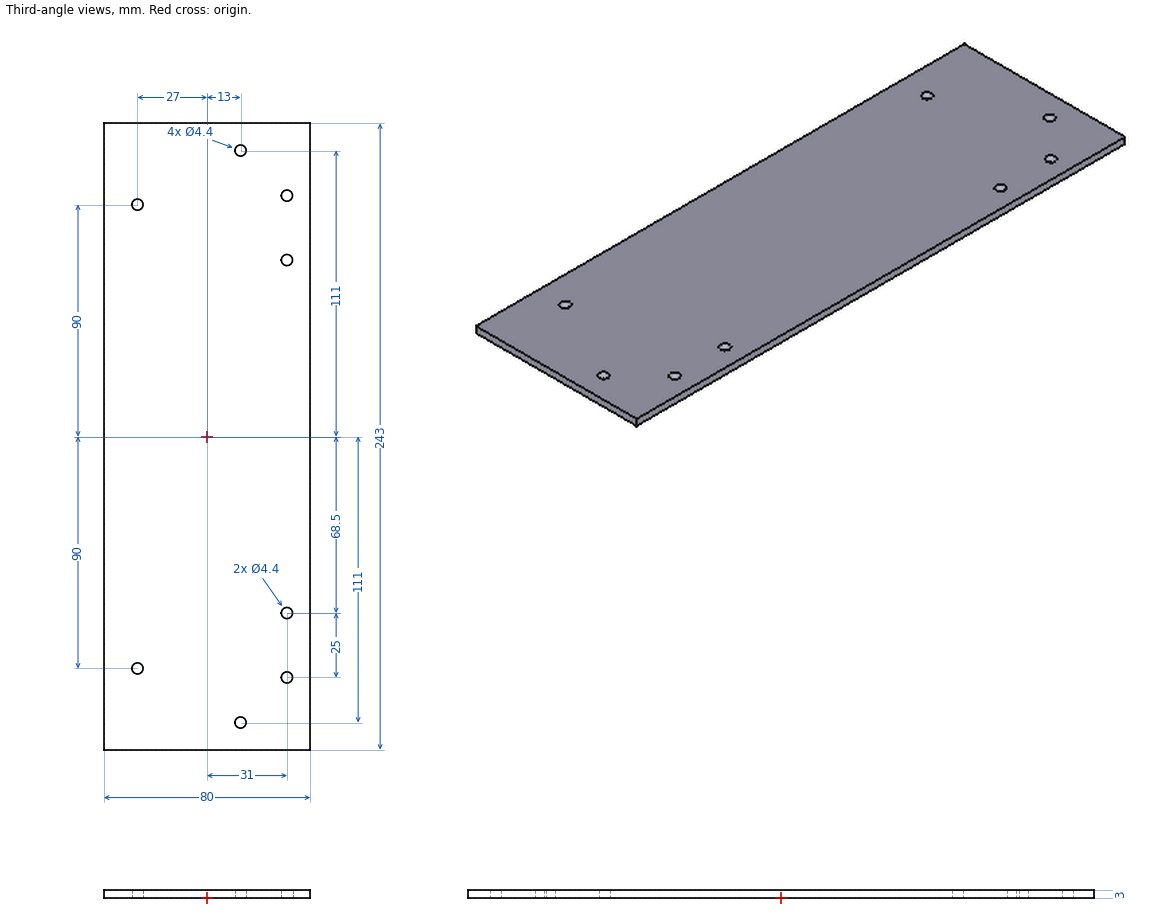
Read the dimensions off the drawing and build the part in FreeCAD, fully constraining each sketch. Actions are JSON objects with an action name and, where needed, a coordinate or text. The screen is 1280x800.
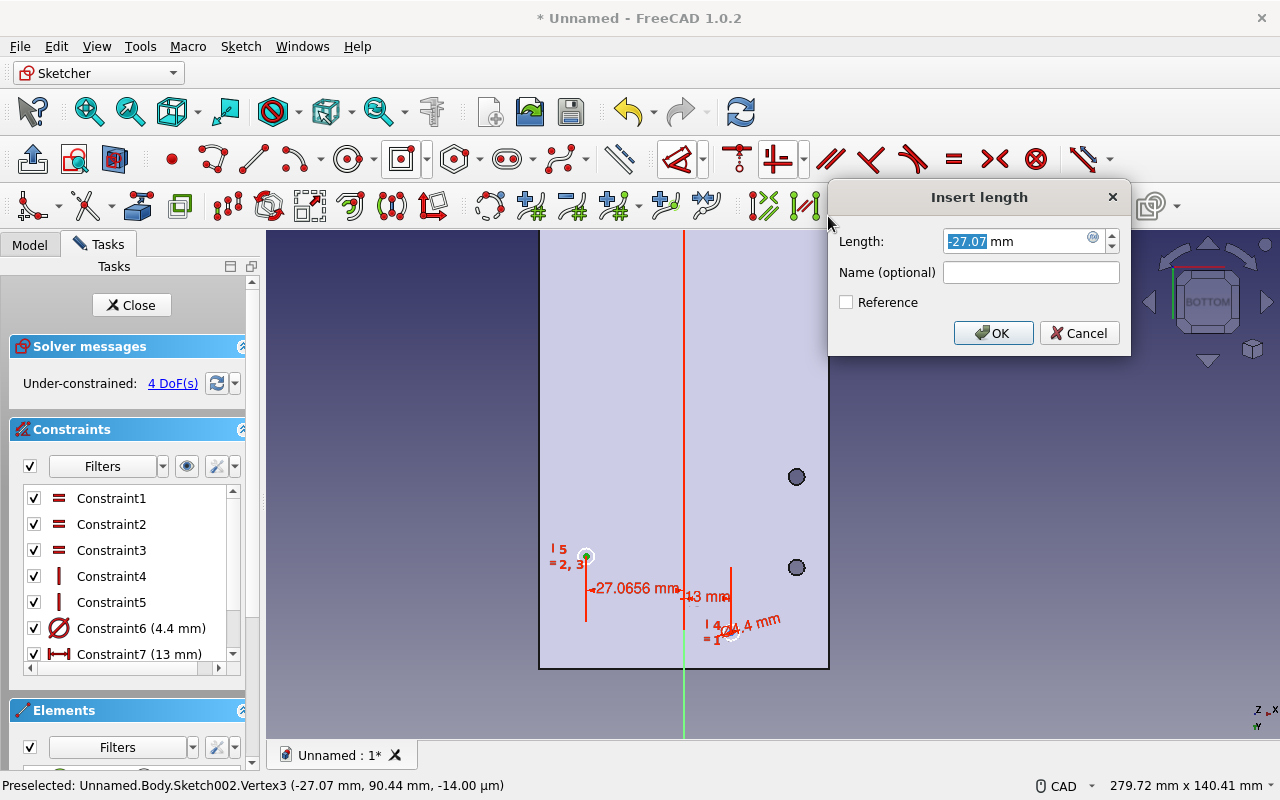
{"action": "type", "text": "-27"}
{"action": "key", "text": "Return"}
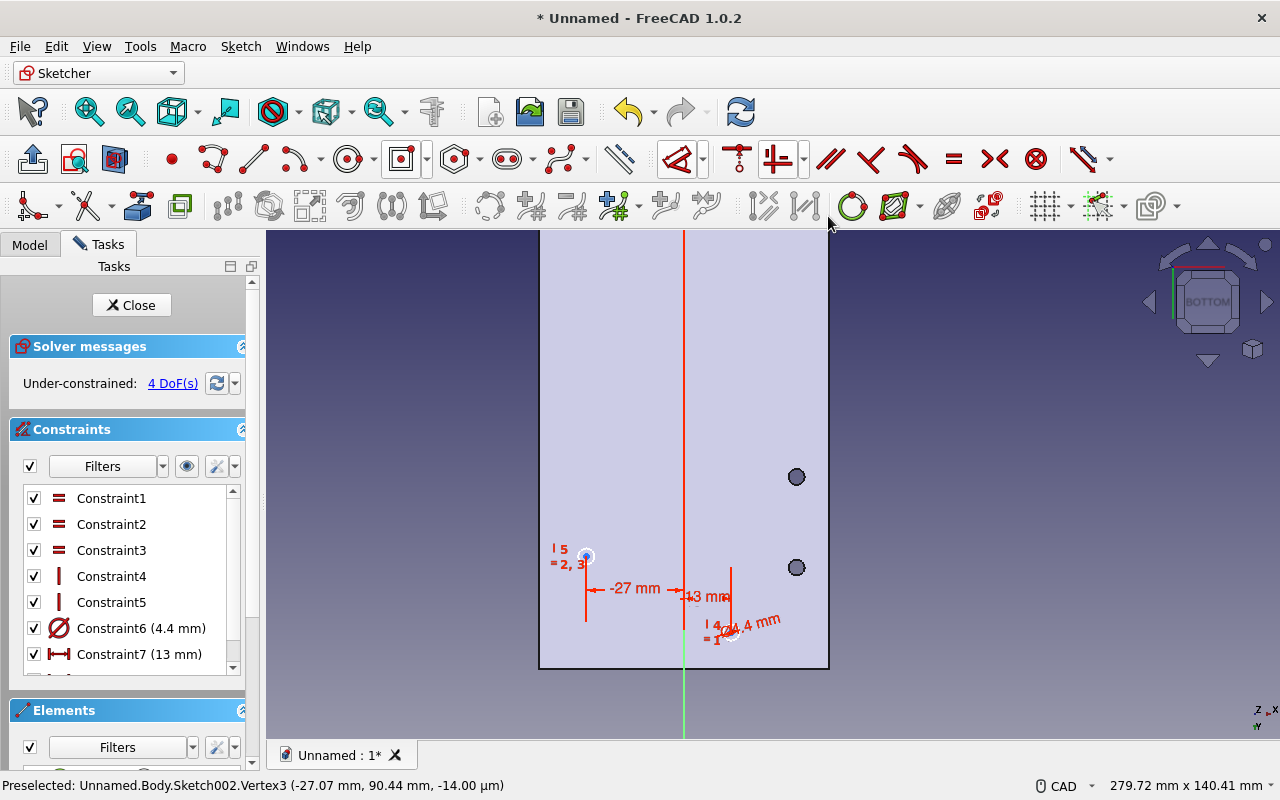
{"action": "left_click", "coordinate": [586, 556]}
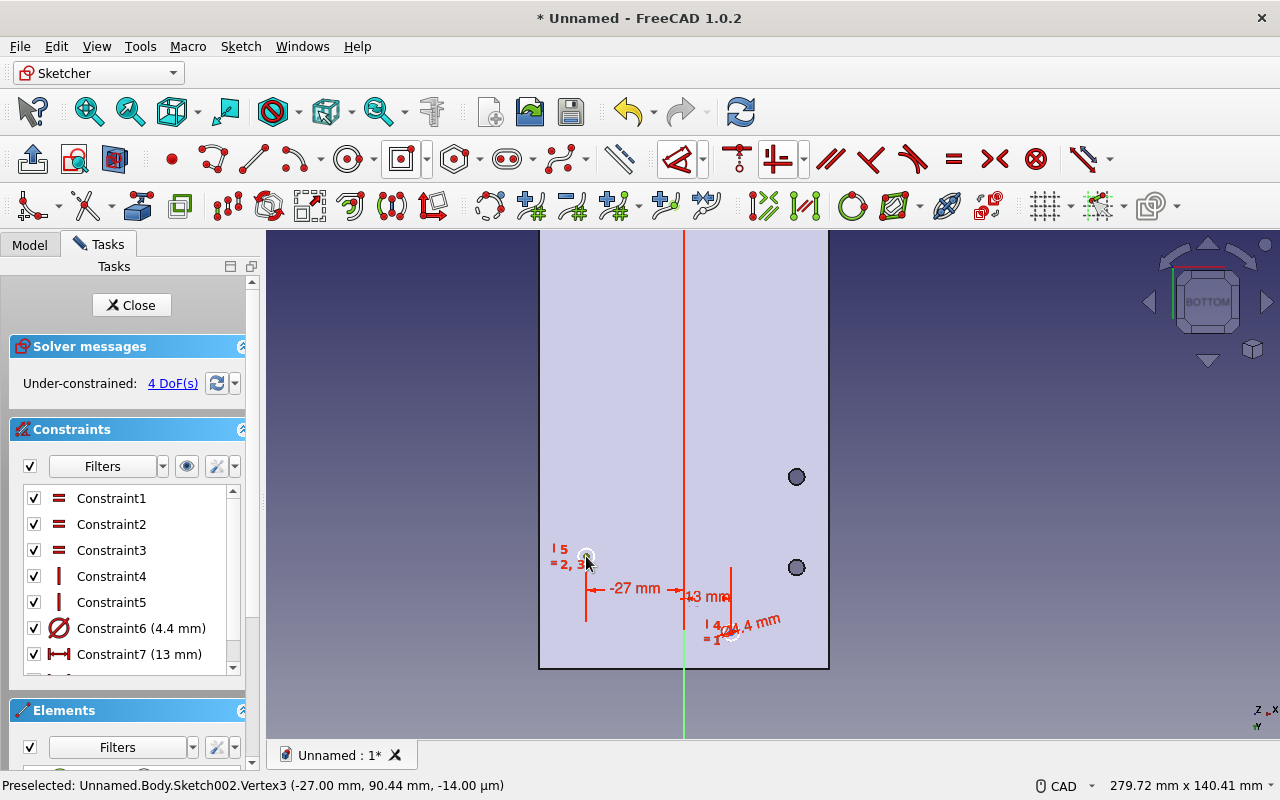
{"action": "key", "text": "i"}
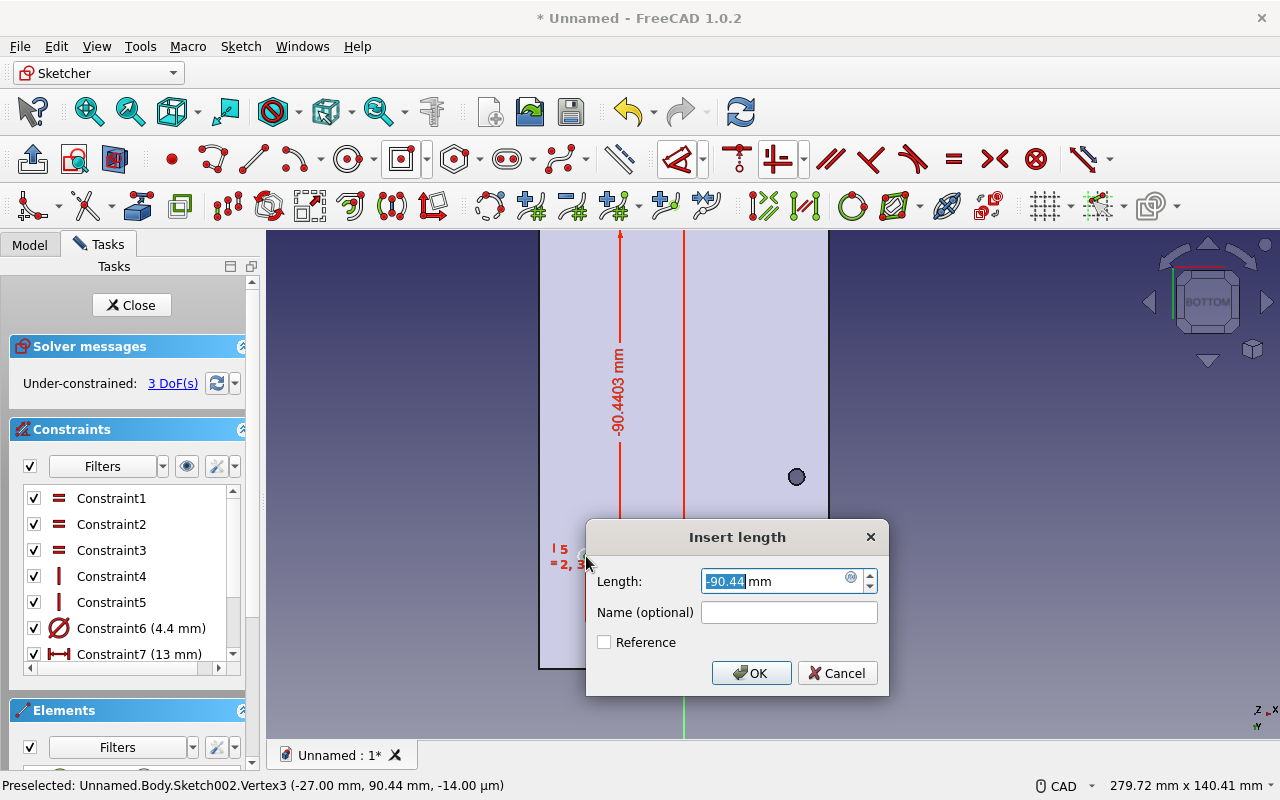
{"action": "type", "text": "-90"}
{"action": "key", "text": "Return"}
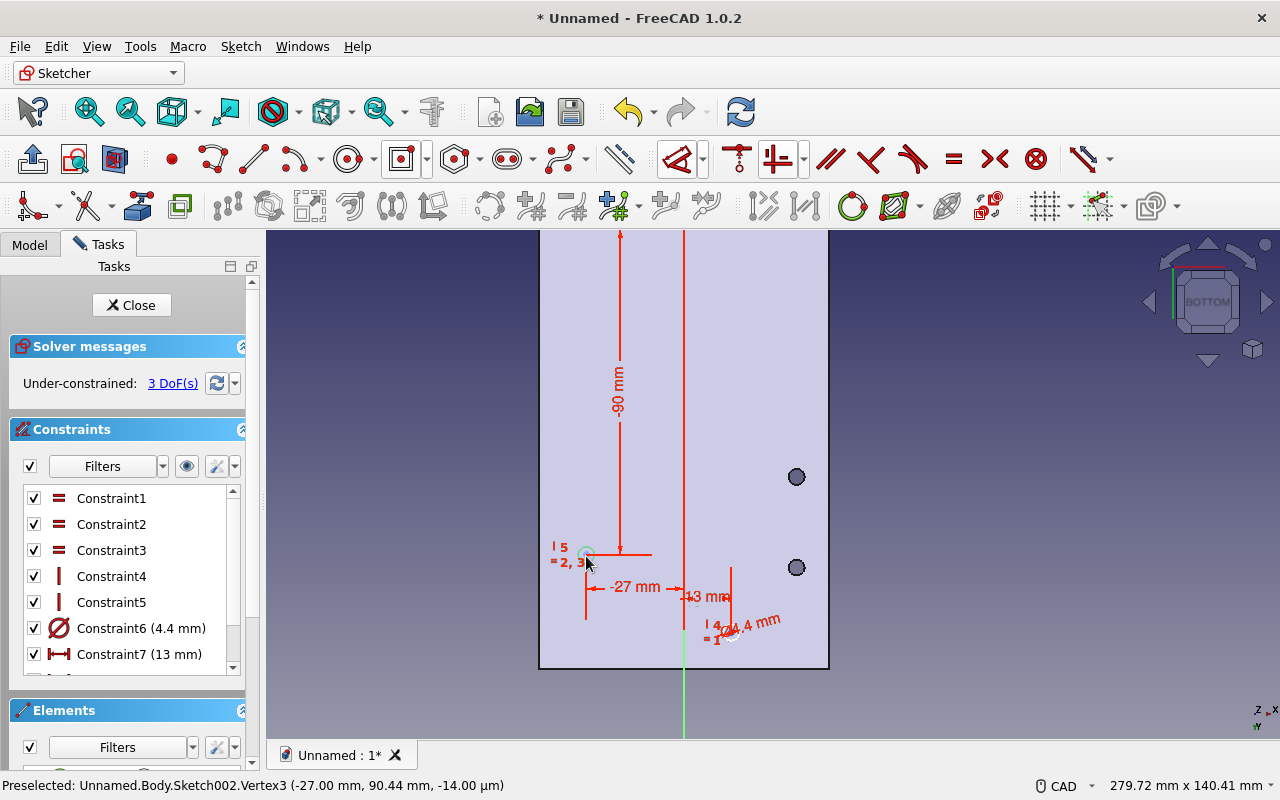
{"action": "scroll", "coordinate": [731, 633], "scroll_direction": "down", "scroll_amount": 5}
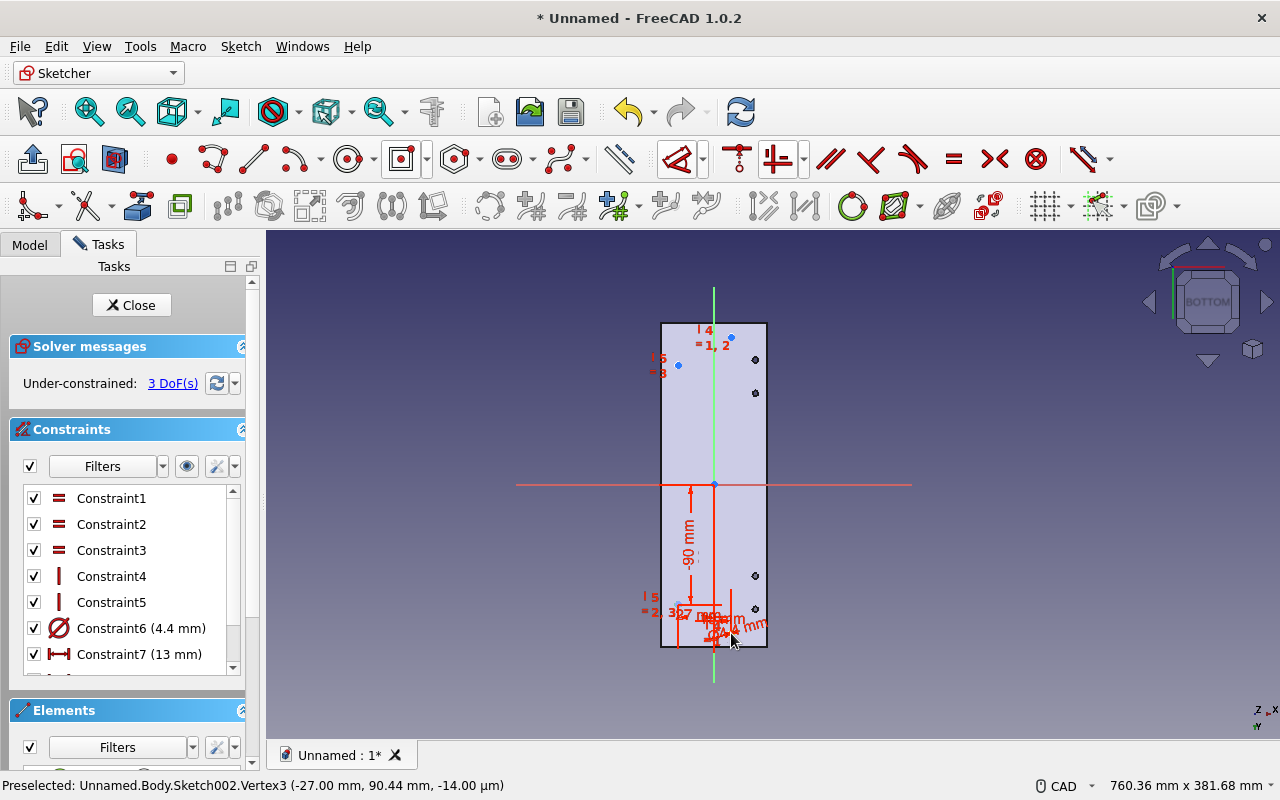
{"action": "left_click", "coordinate": [678, 365]}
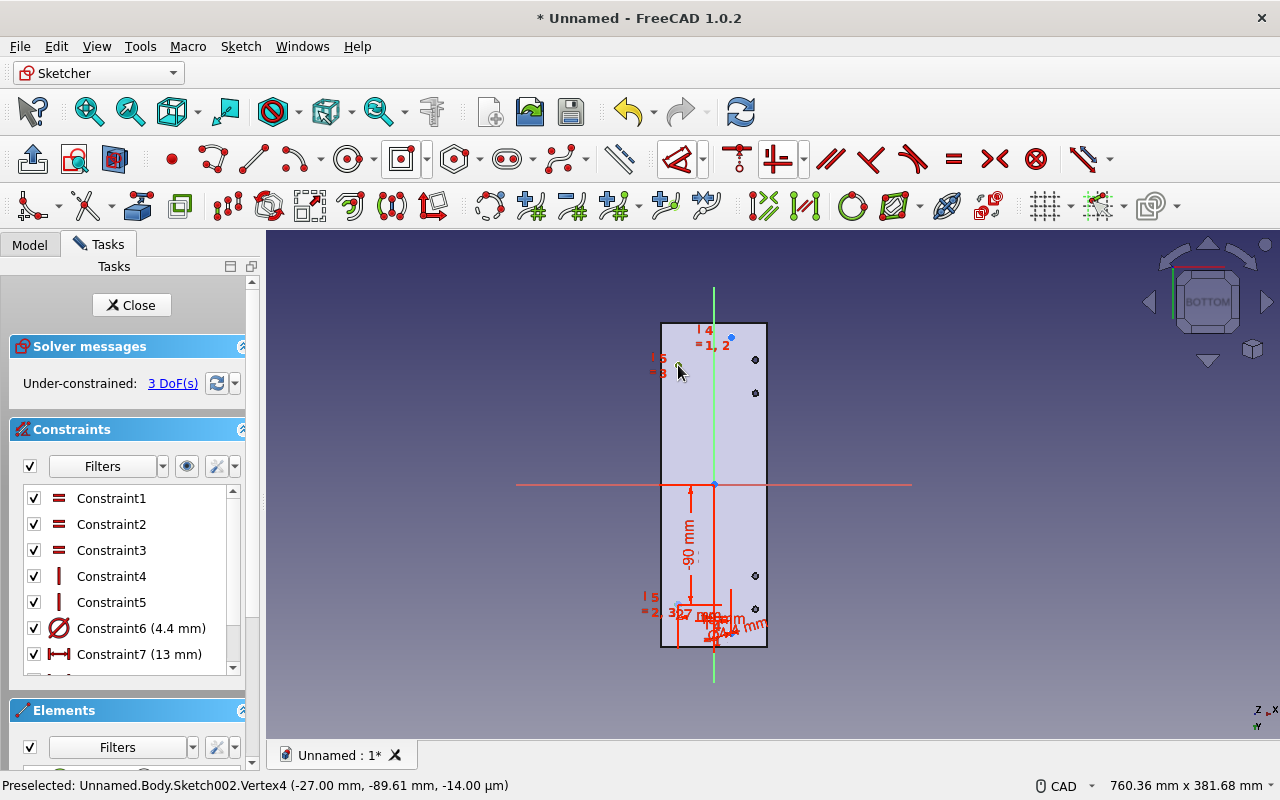
{"action": "key", "text": "i"}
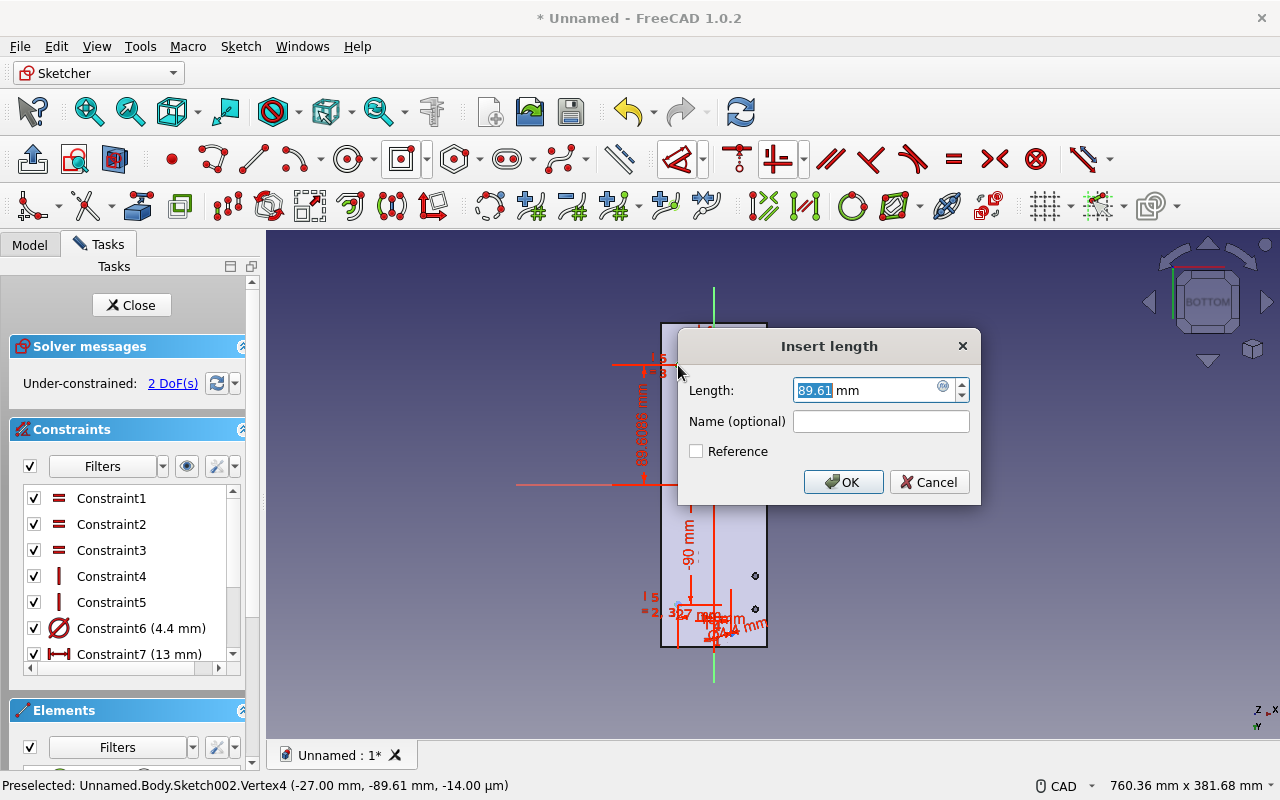
{"action": "type", "text": "90"}
{"action": "key", "text": "Return"}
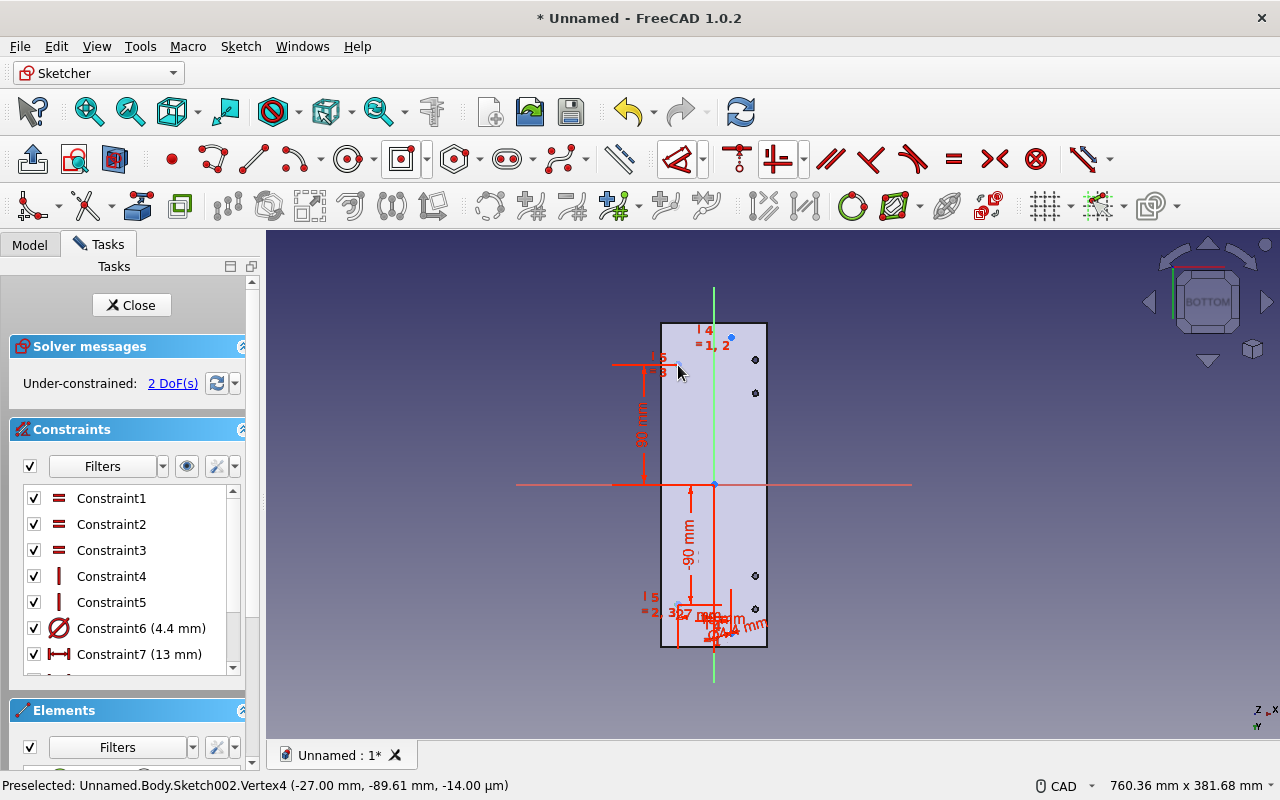
{"action": "left_click", "coordinate": [731, 633]}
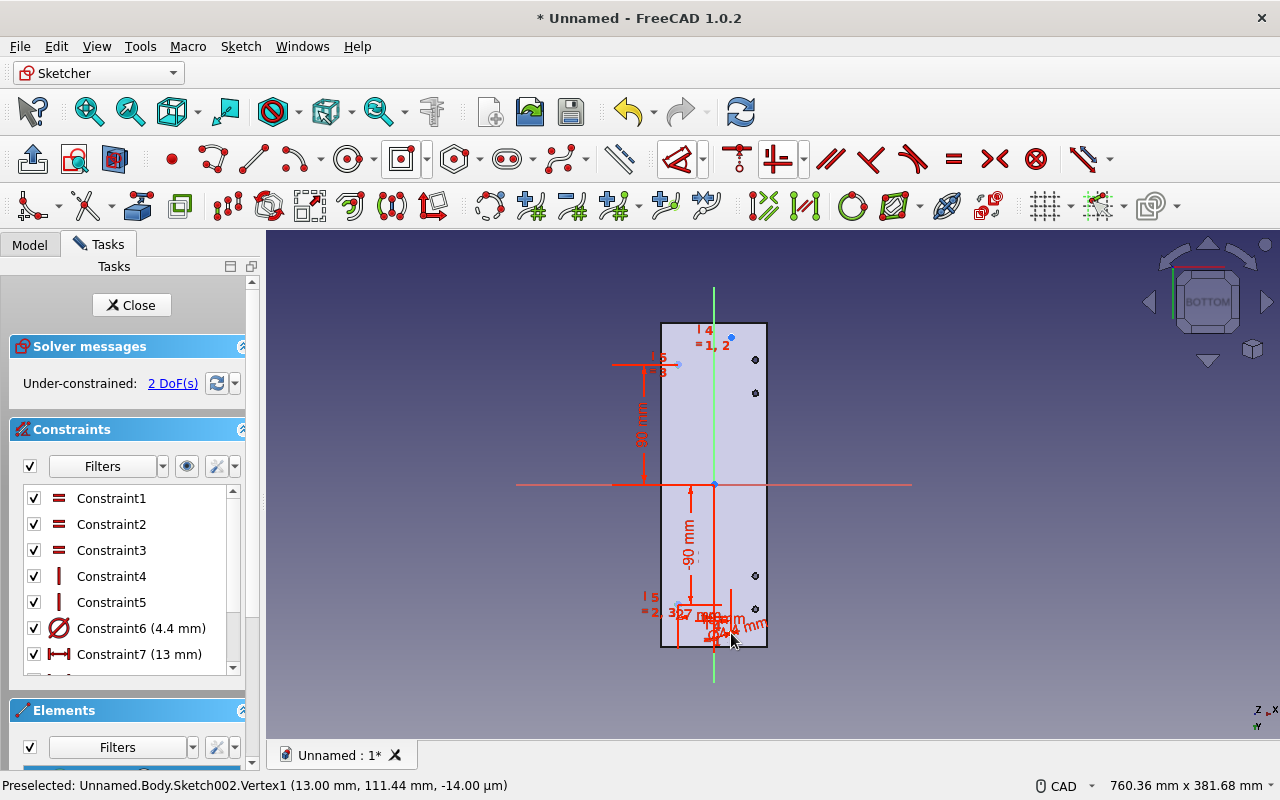
{"action": "left_click", "coordinate": [702, 160]}